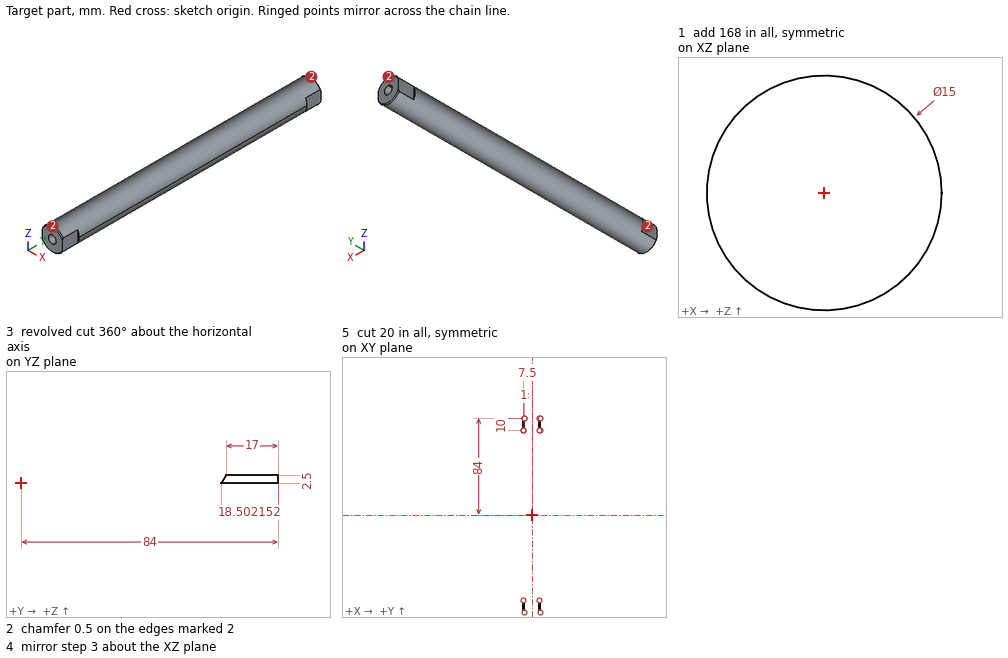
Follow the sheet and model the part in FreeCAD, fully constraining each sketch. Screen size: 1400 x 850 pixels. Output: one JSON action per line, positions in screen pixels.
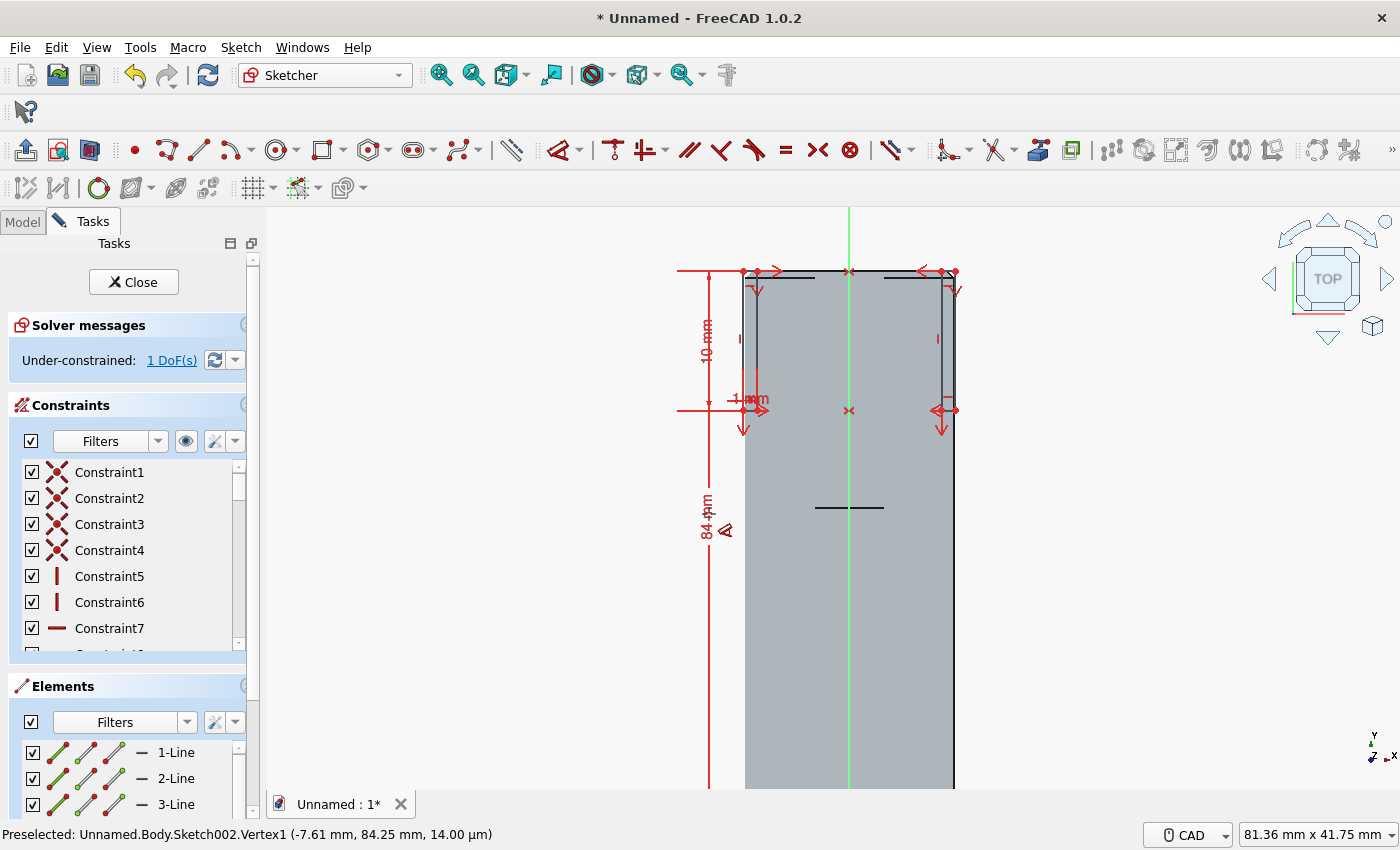
{"action": "left_click", "coordinate": [743, 271]}
{"action": "left_click", "coordinate": [796, 237]}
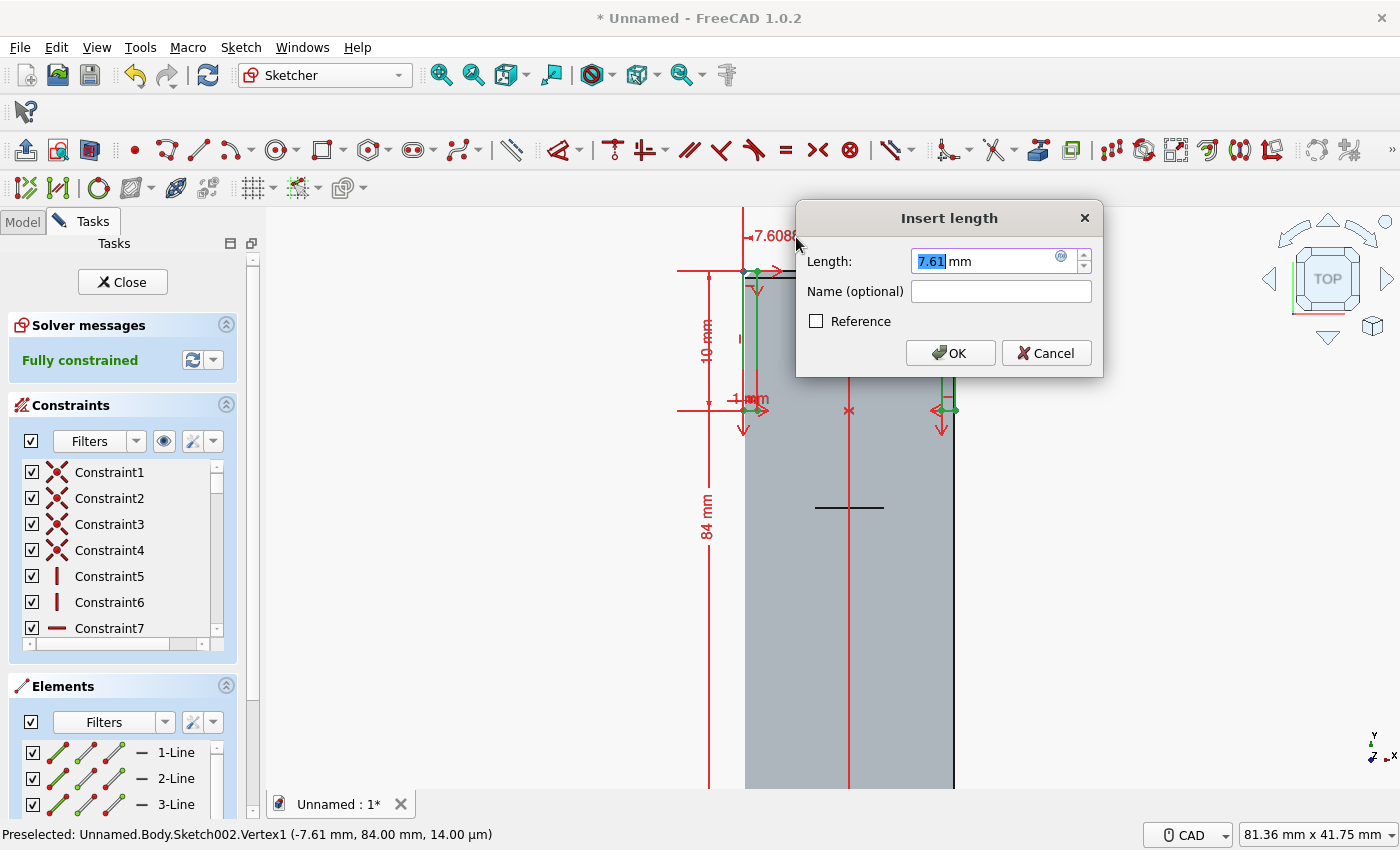
{"action": "type", "text": "7.5"}
{"action": "key", "text": "Return"}
{"action": "key", "text": "Escape"}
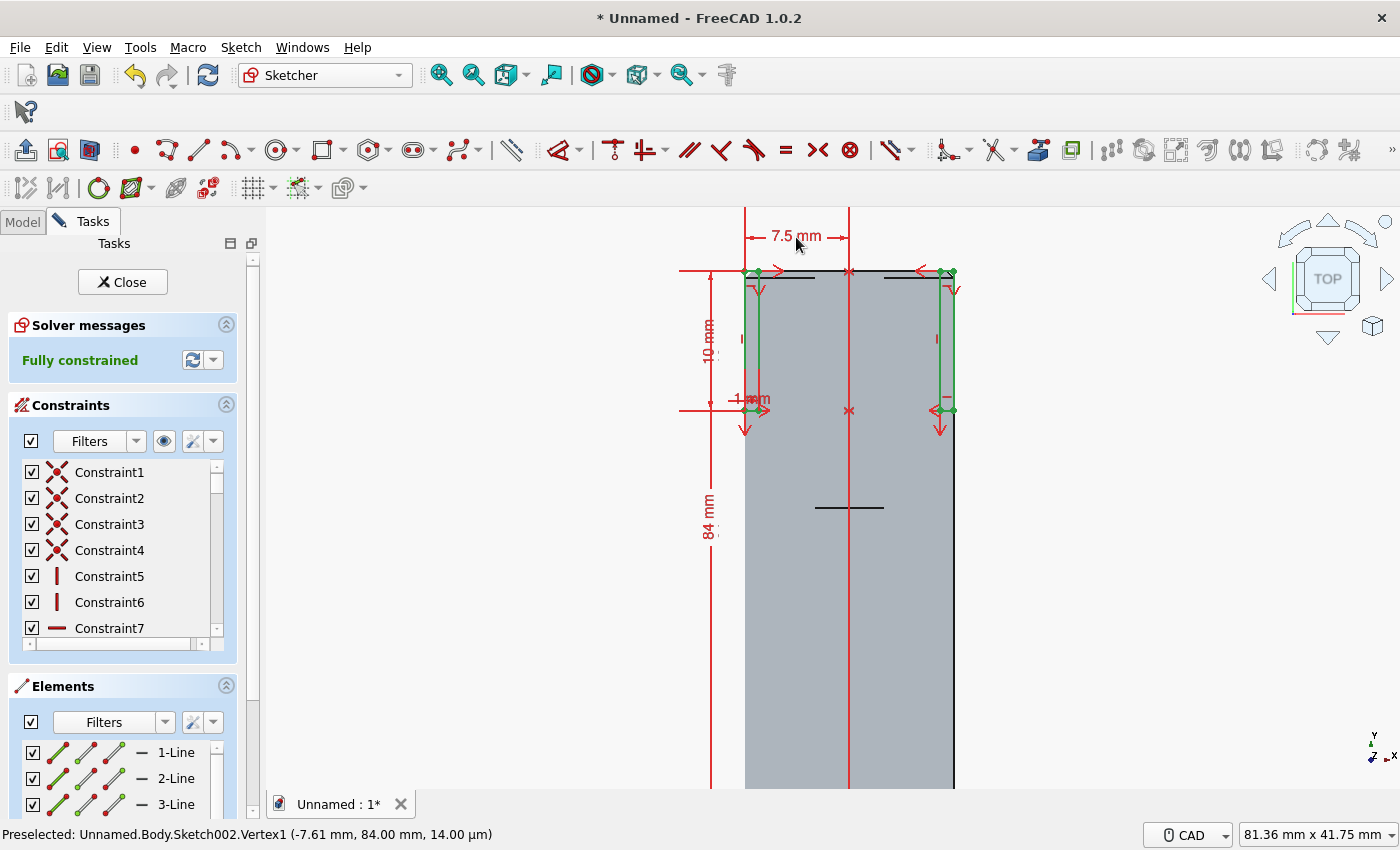
{"action": "left_click", "coordinate": [123, 282]}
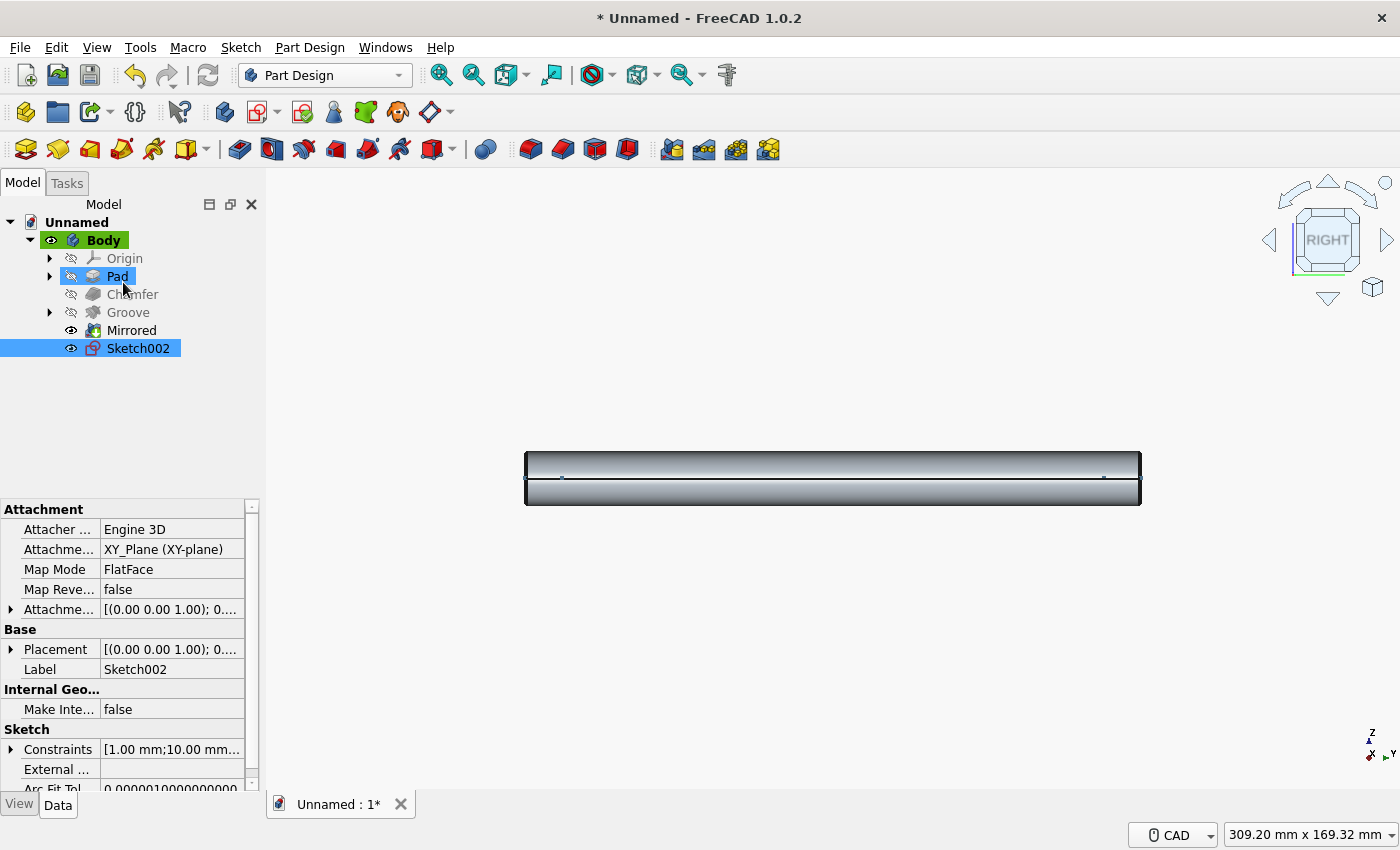
{"action": "left_click", "coordinate": [240, 150]}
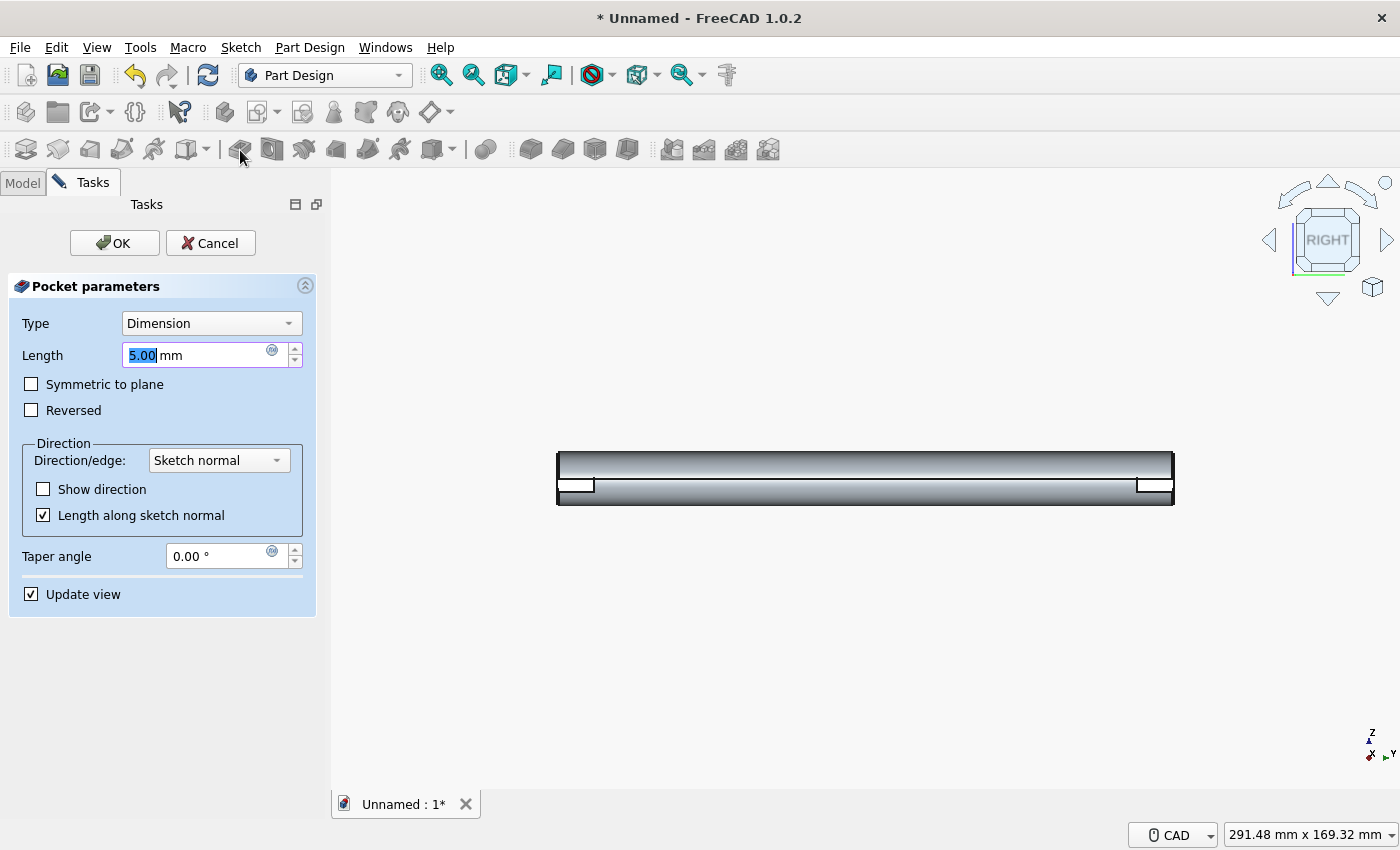
{"action": "type", "text": "20"}
{"action": "key", "text": "Tab"}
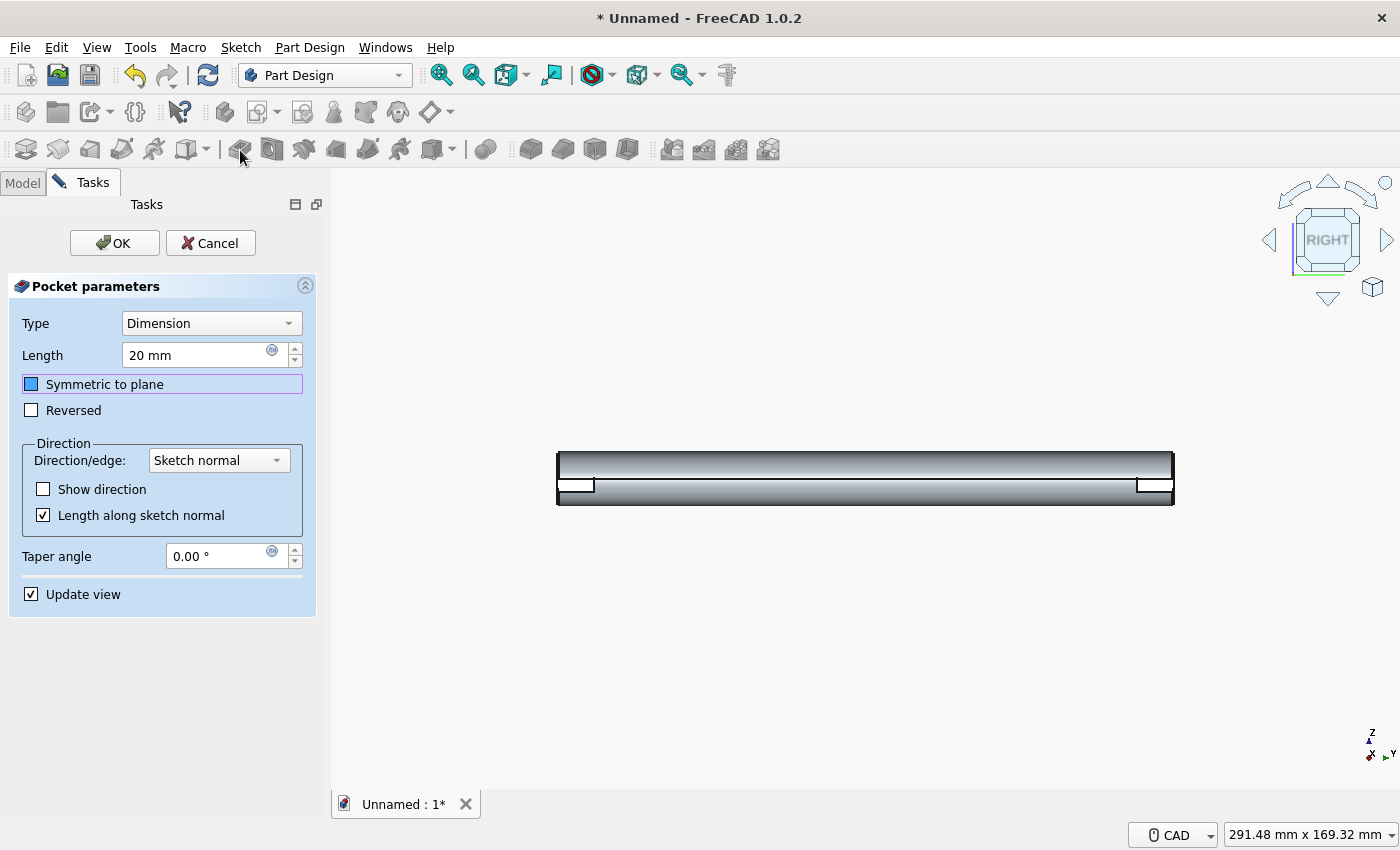
{"action": "left_click", "coordinate": [30, 384]}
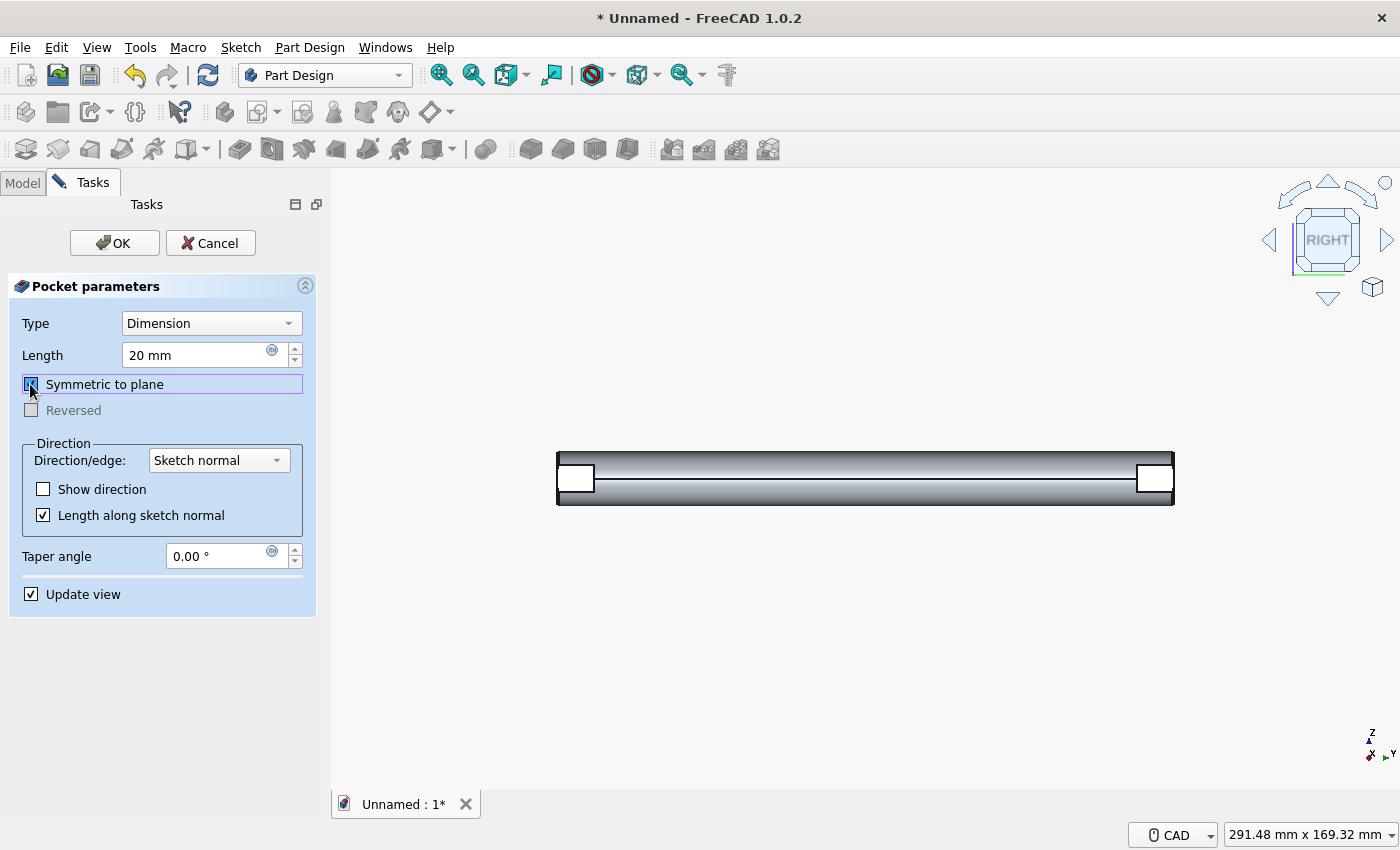
{"action": "left_click", "coordinate": [115, 243]}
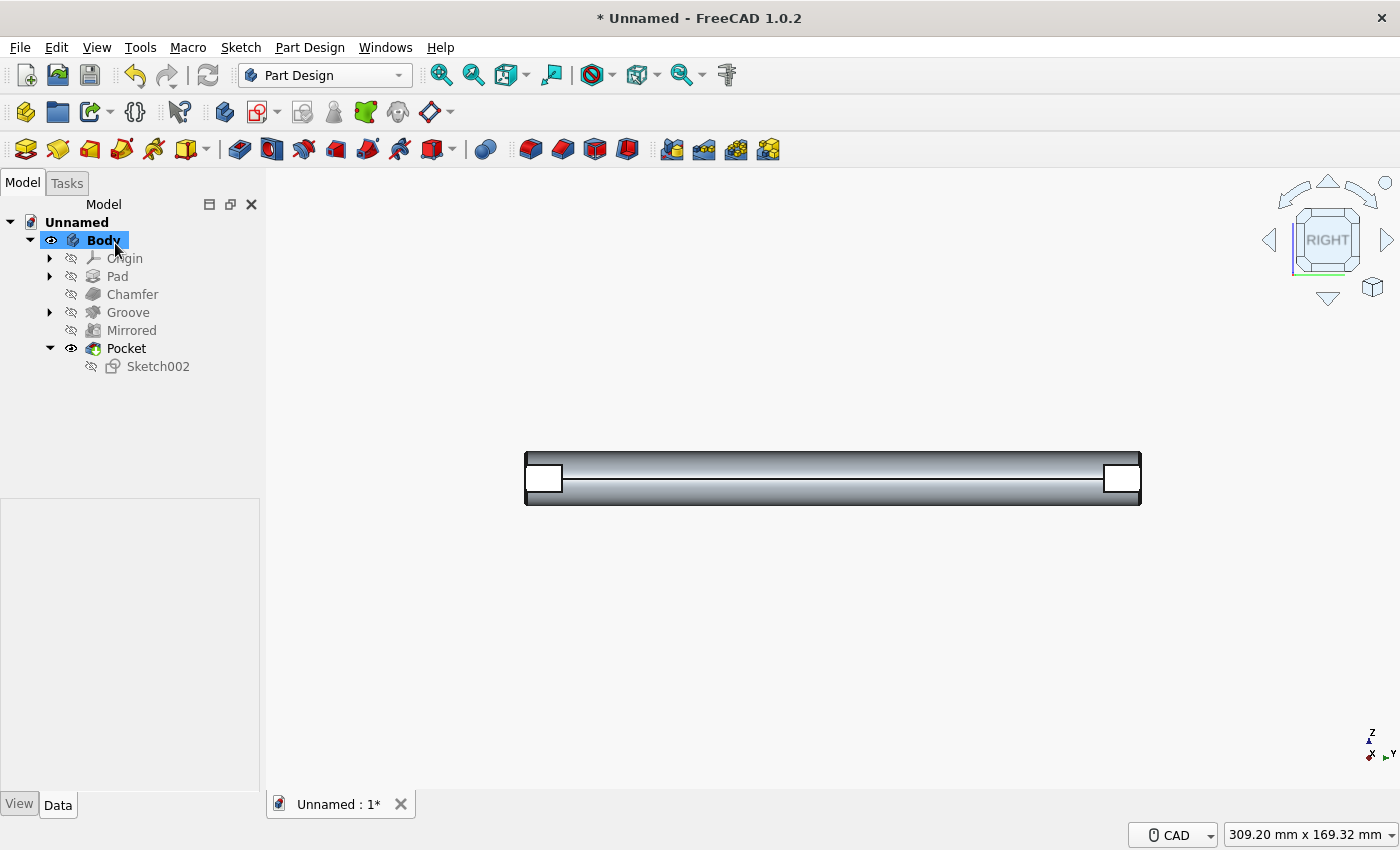
{"action": "key", "text": "0"}